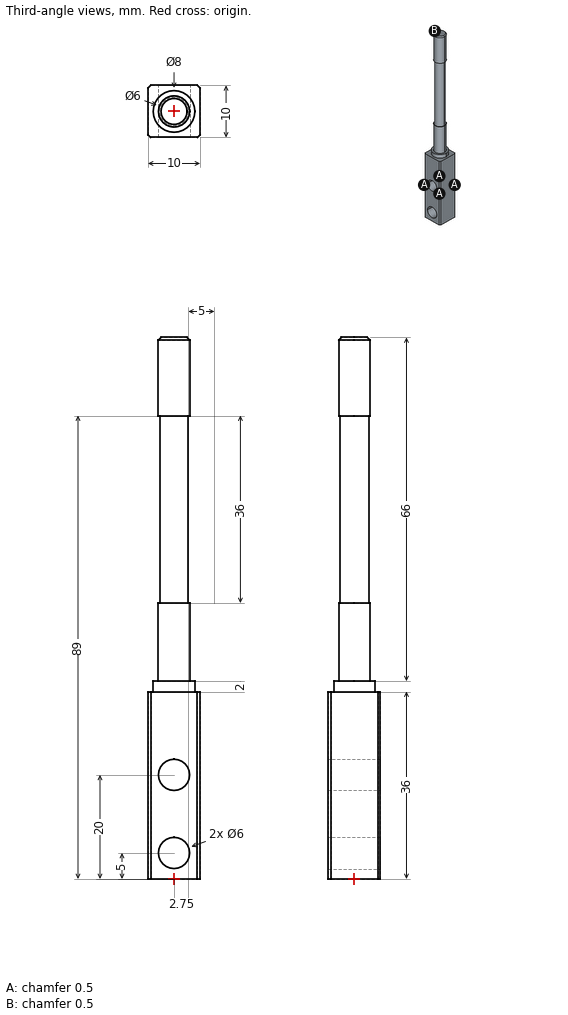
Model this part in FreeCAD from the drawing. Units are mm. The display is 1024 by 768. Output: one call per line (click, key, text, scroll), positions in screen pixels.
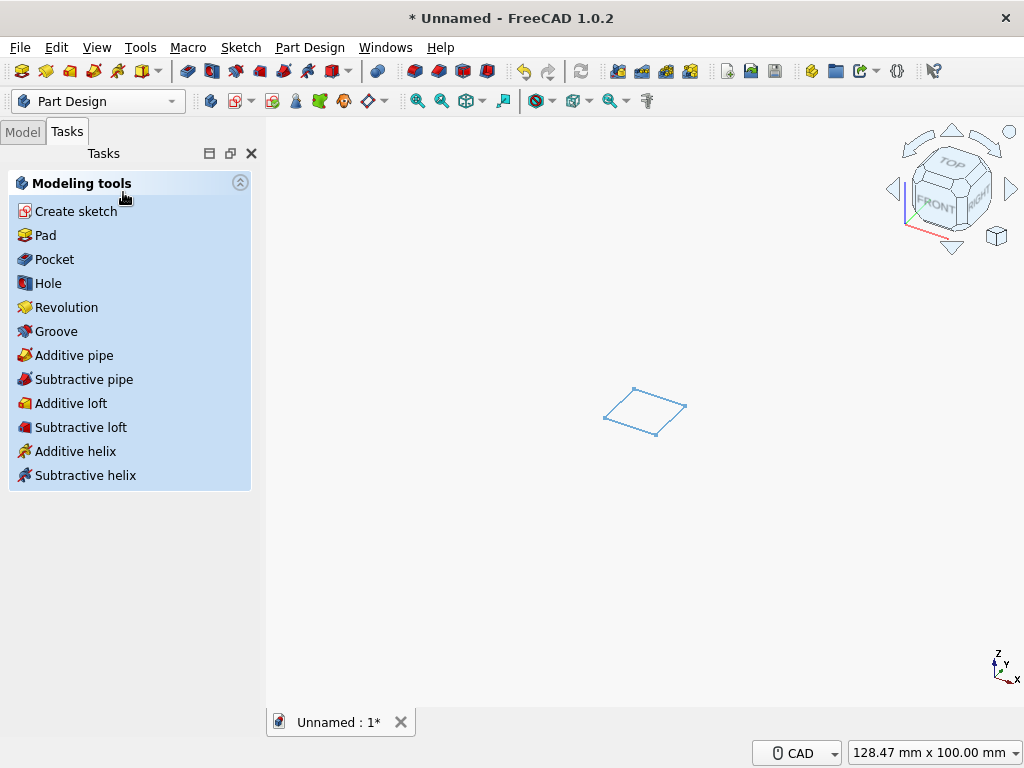
click(22, 72)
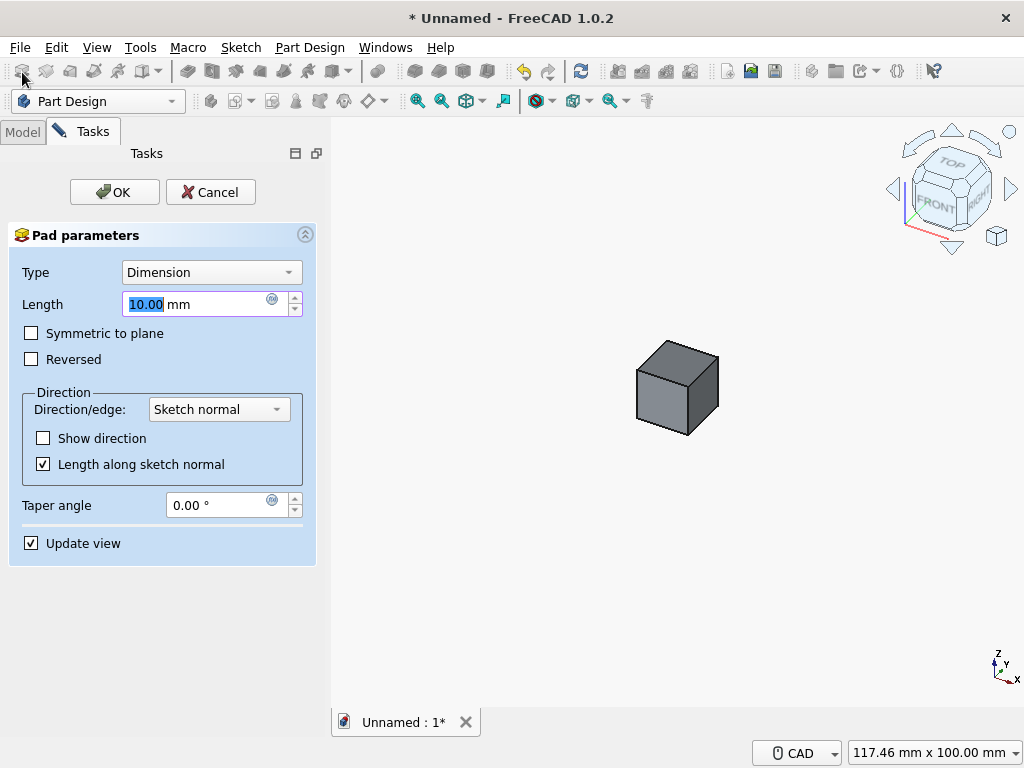
text(36)
key(Tab)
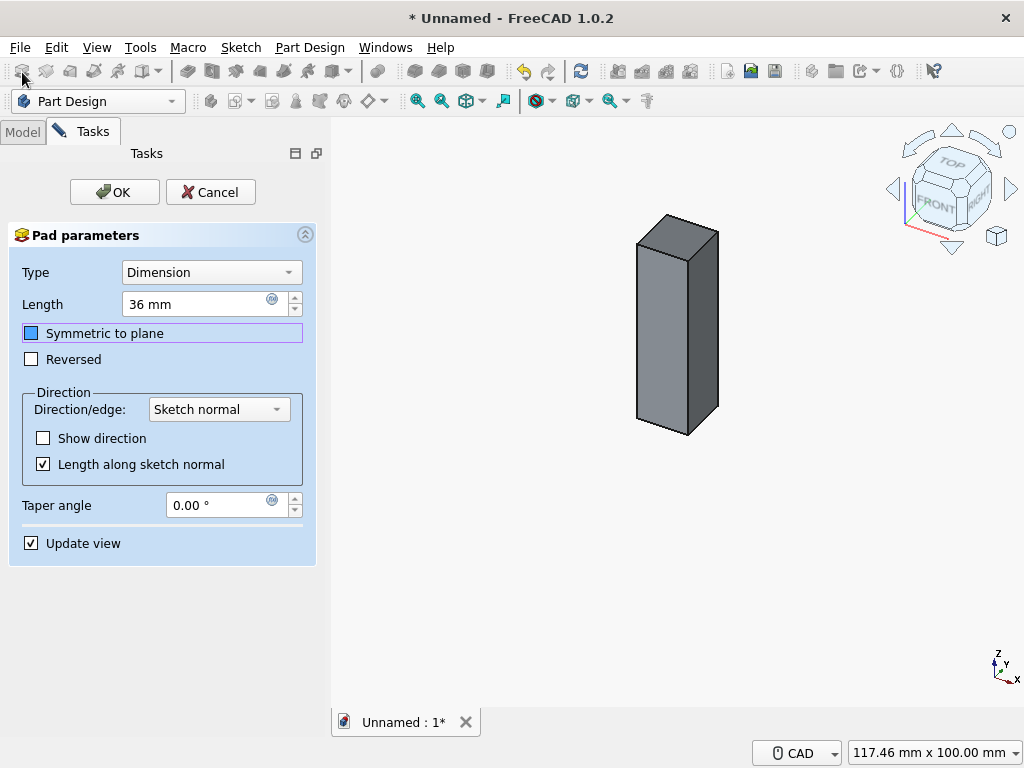
click(115, 192)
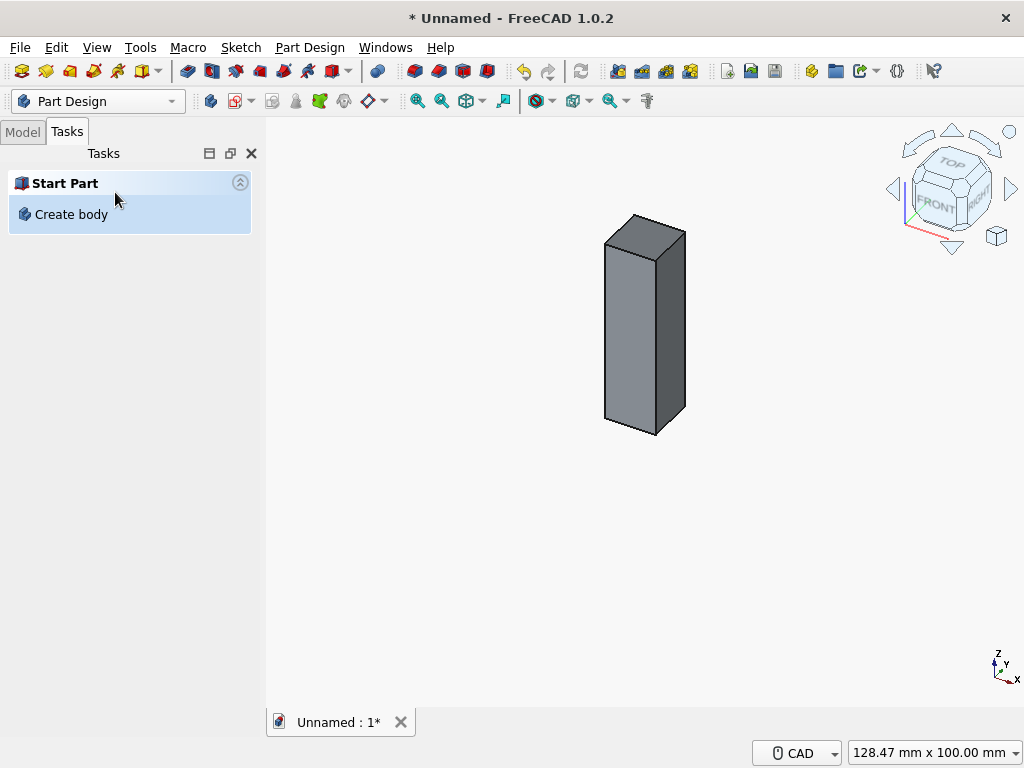
key(v)
key(f)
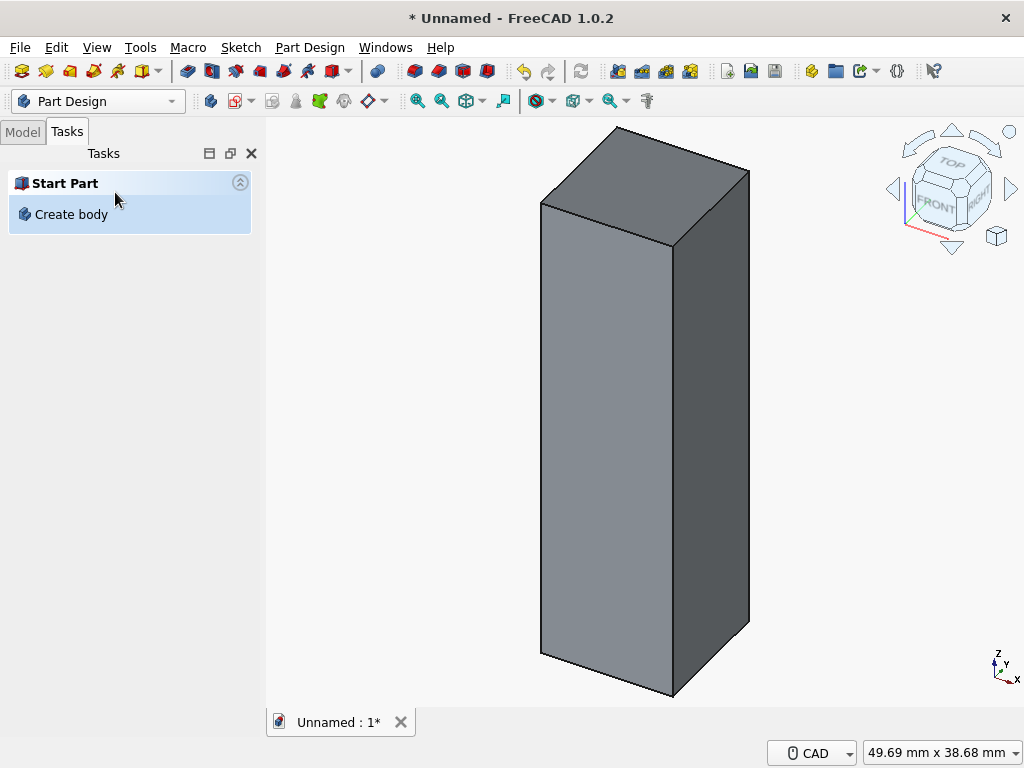
click(645, 186)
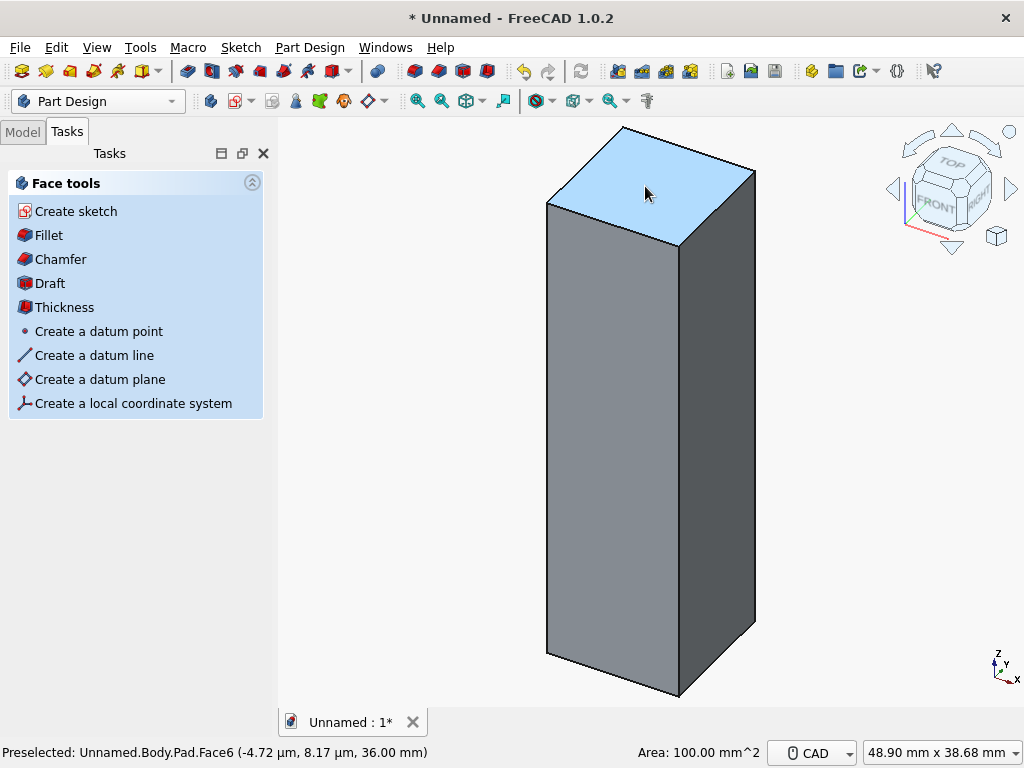
click(236, 102)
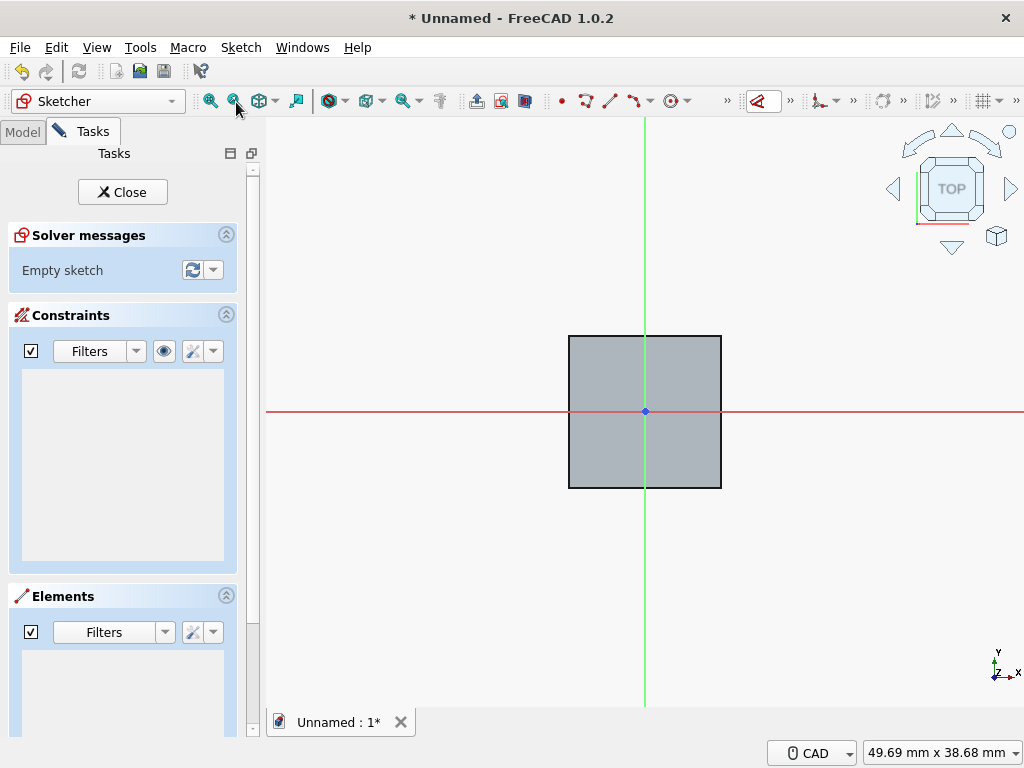
scroll(675, 412, up, 6)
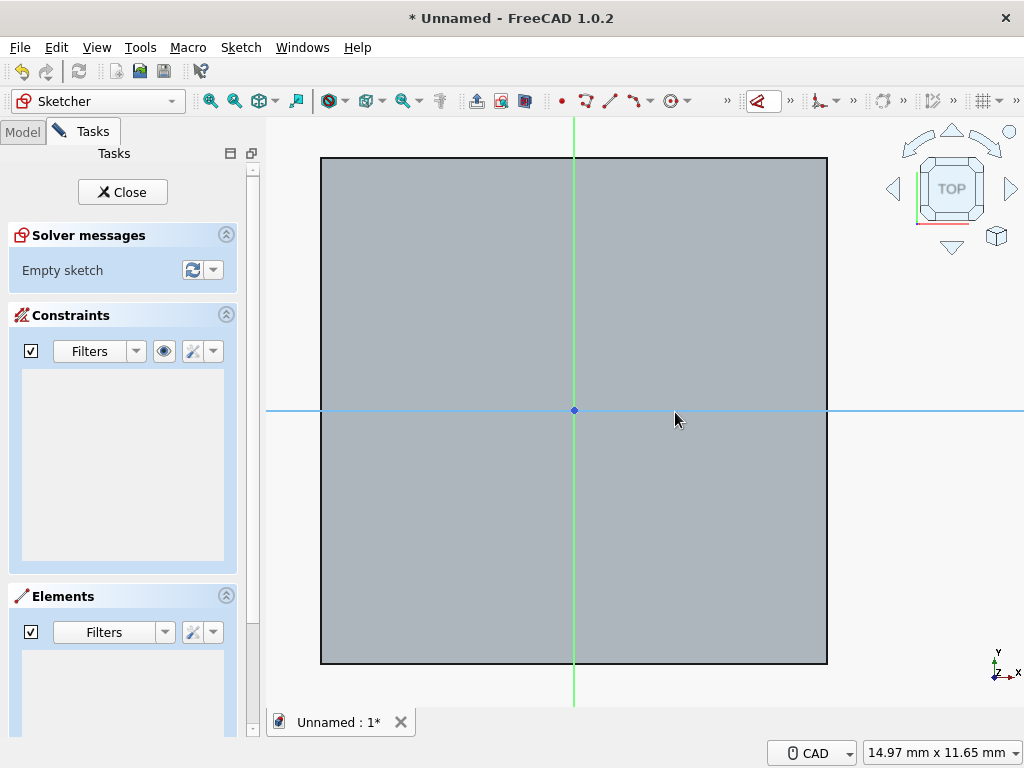
click(672, 102)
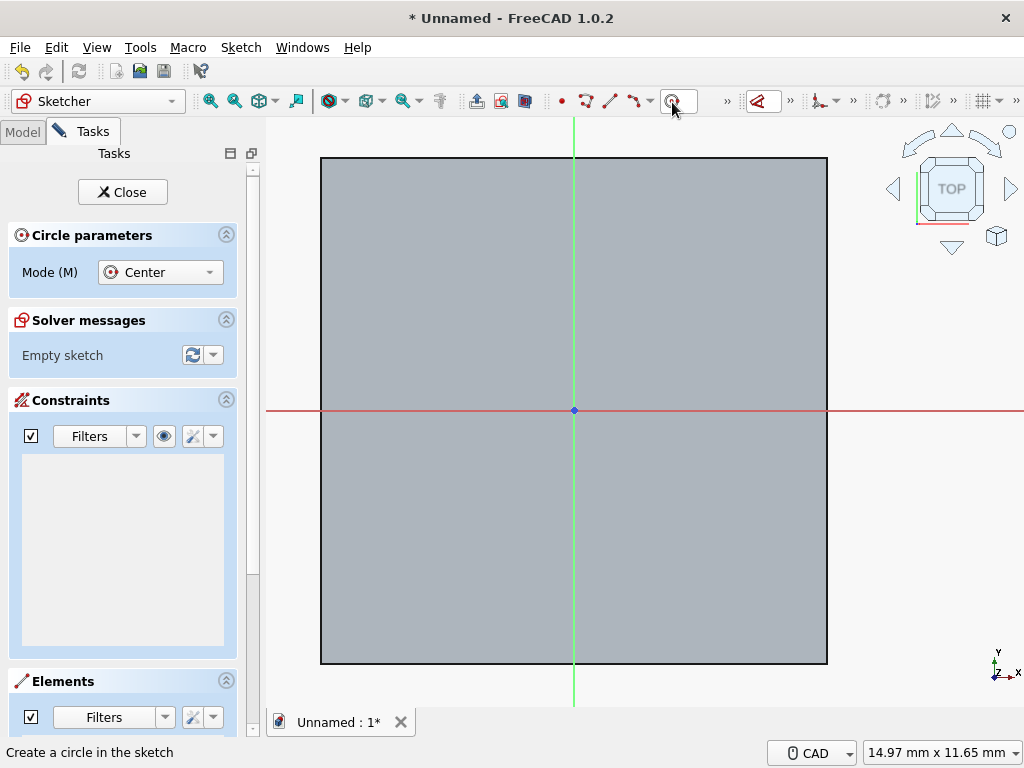
click(574, 411)
click(717, 268)
key(Escape)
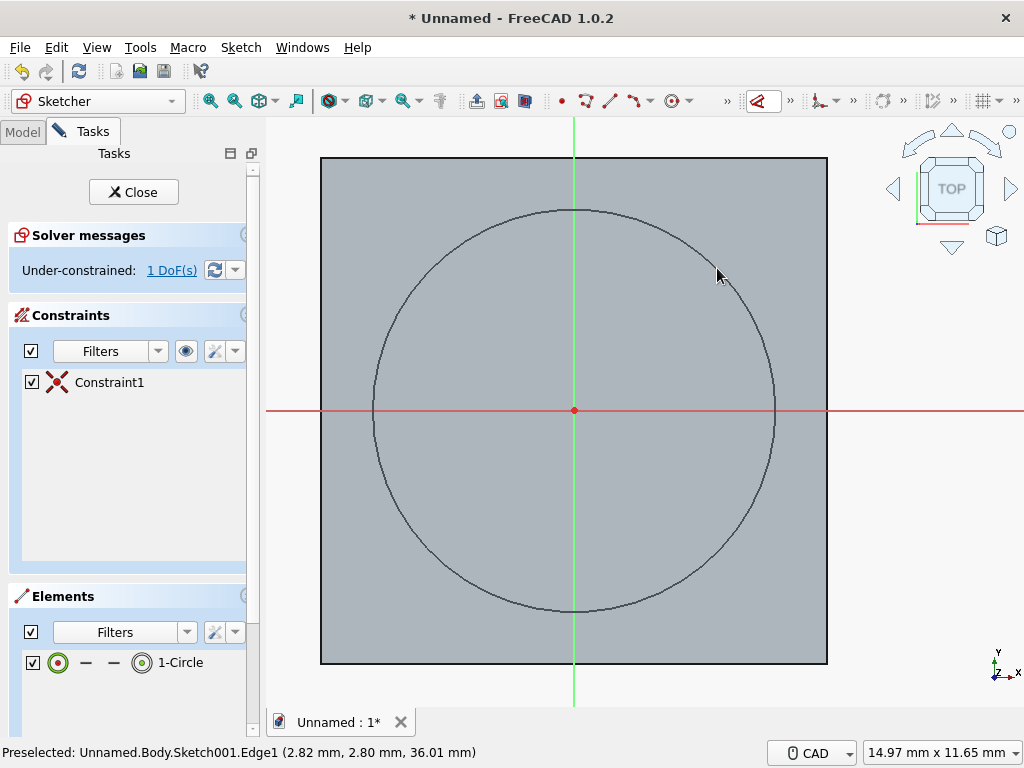
key(d)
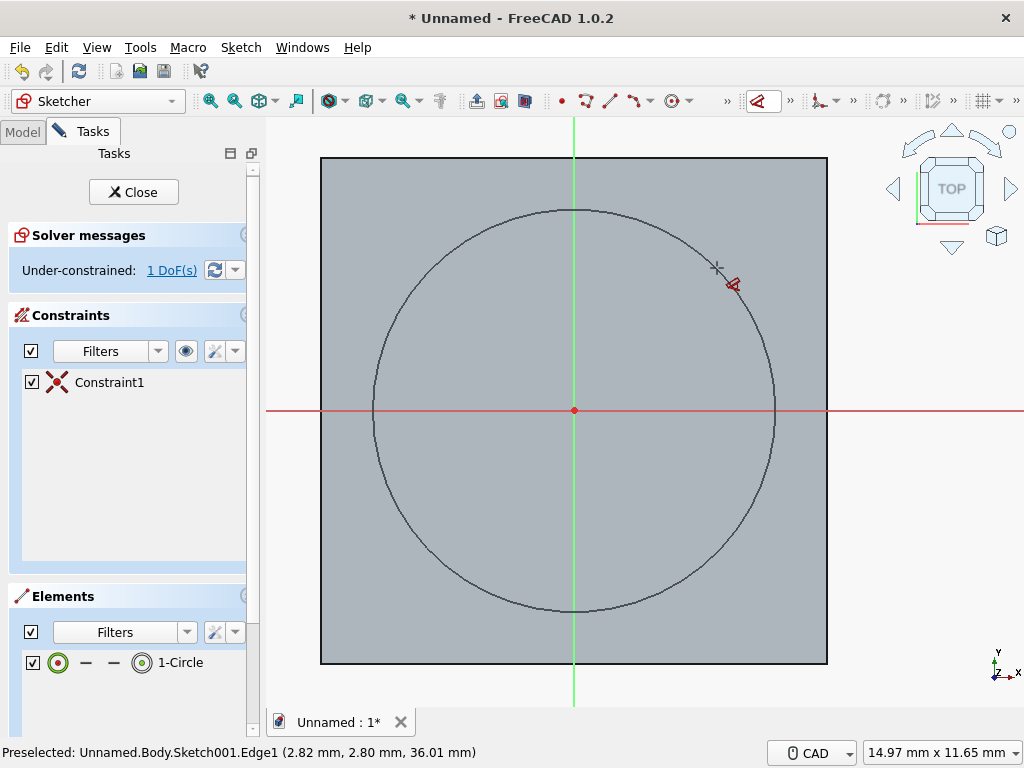
click(716, 268)
click(739, 245)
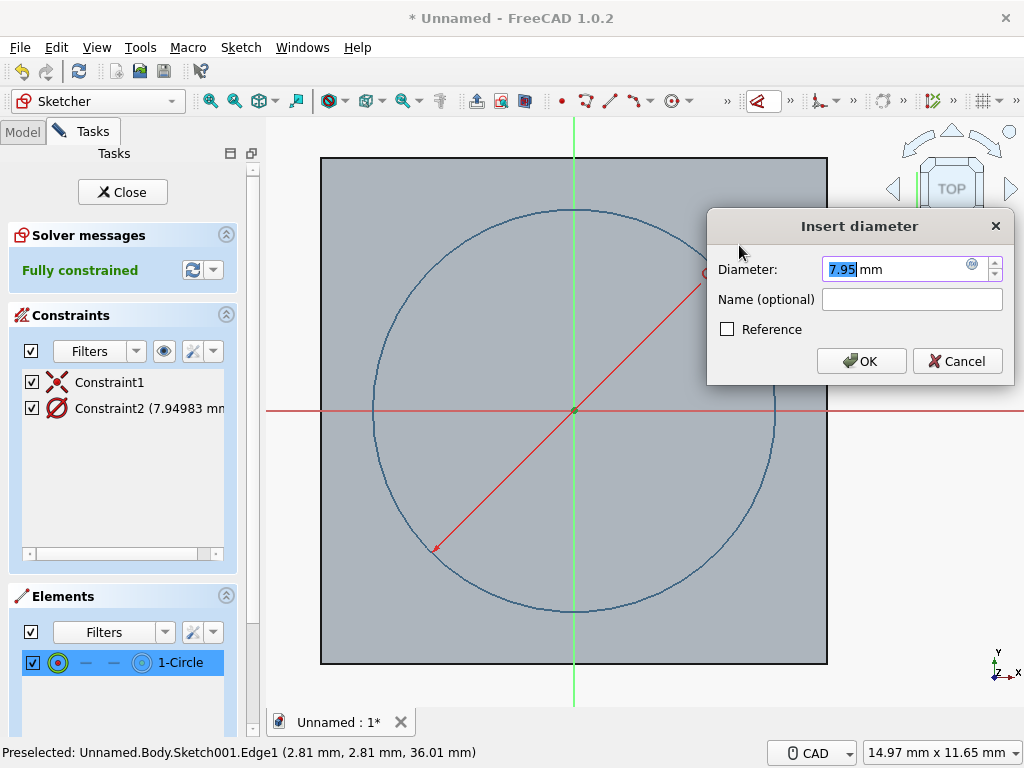
text(8)
key(Return)
key(Escape)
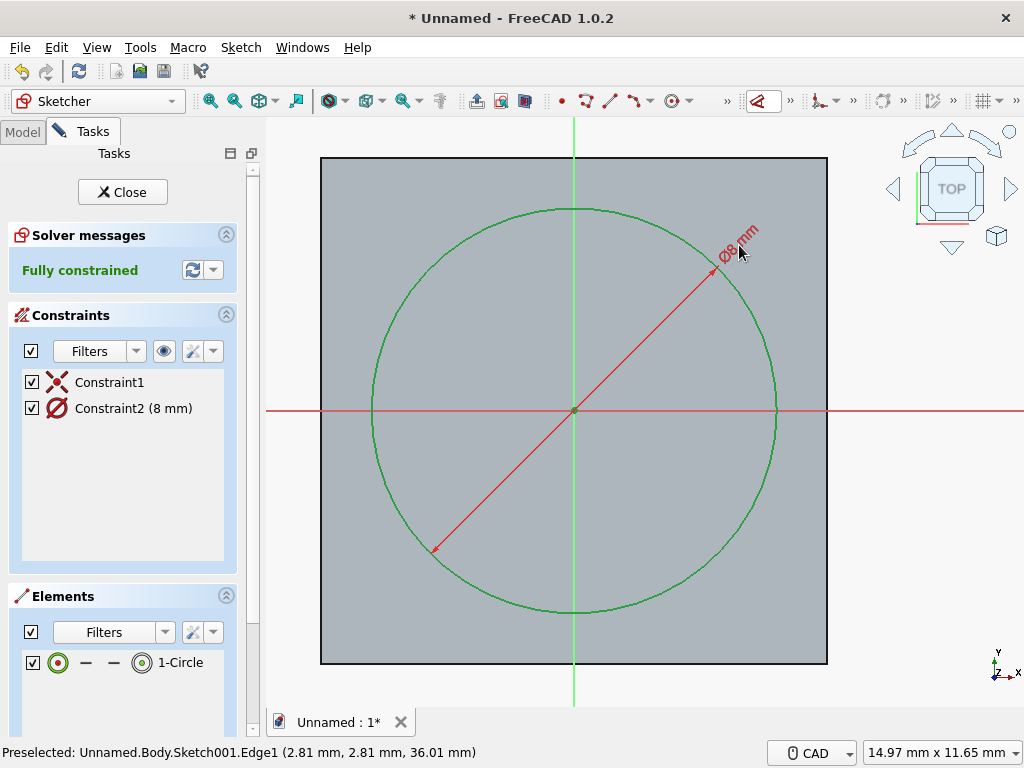
click(123, 192)